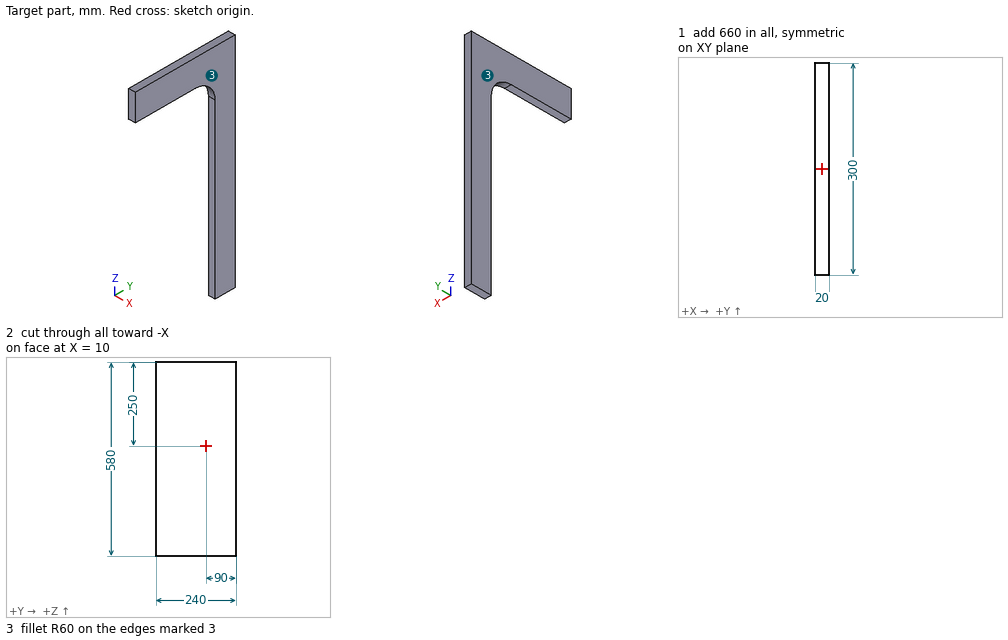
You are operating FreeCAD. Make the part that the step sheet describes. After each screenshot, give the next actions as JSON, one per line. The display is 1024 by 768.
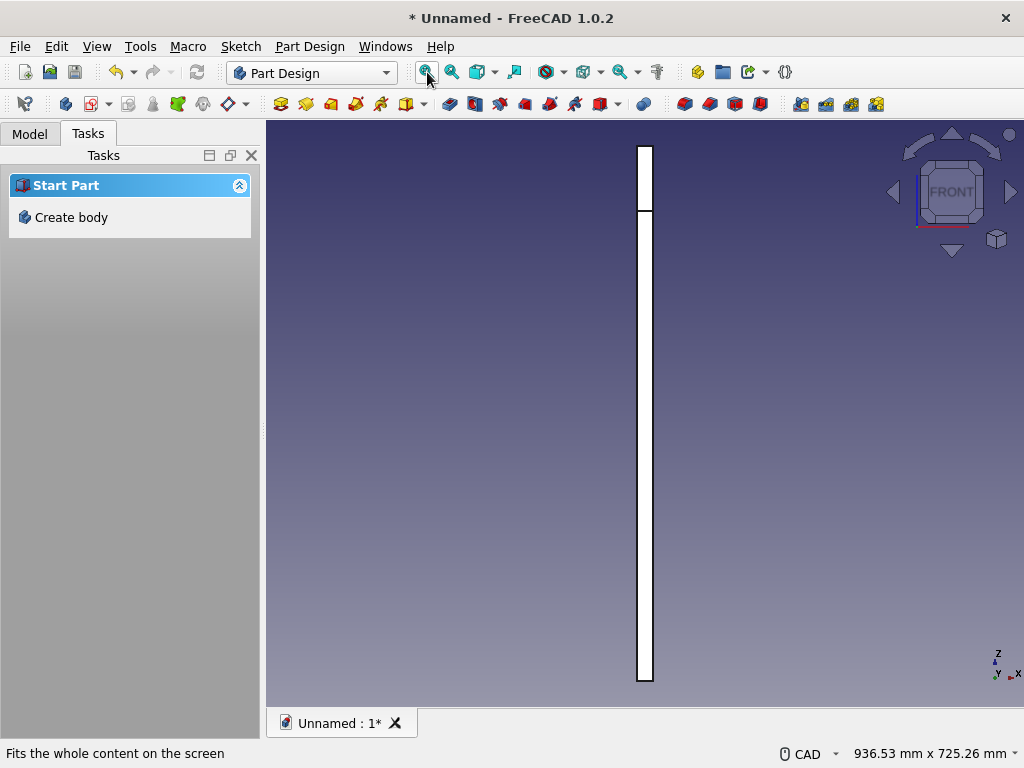
{"action": "key", "text": "3"}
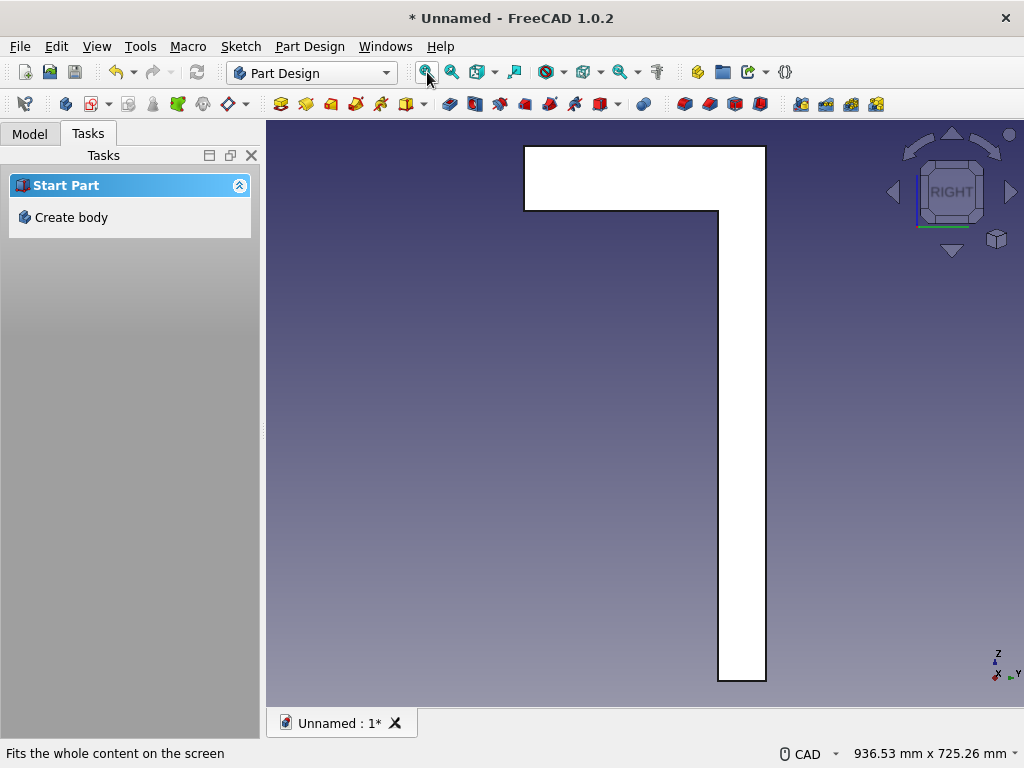
{"action": "scroll", "coordinate": [718, 210], "scroll_direction": "up", "scroll_amount": 5}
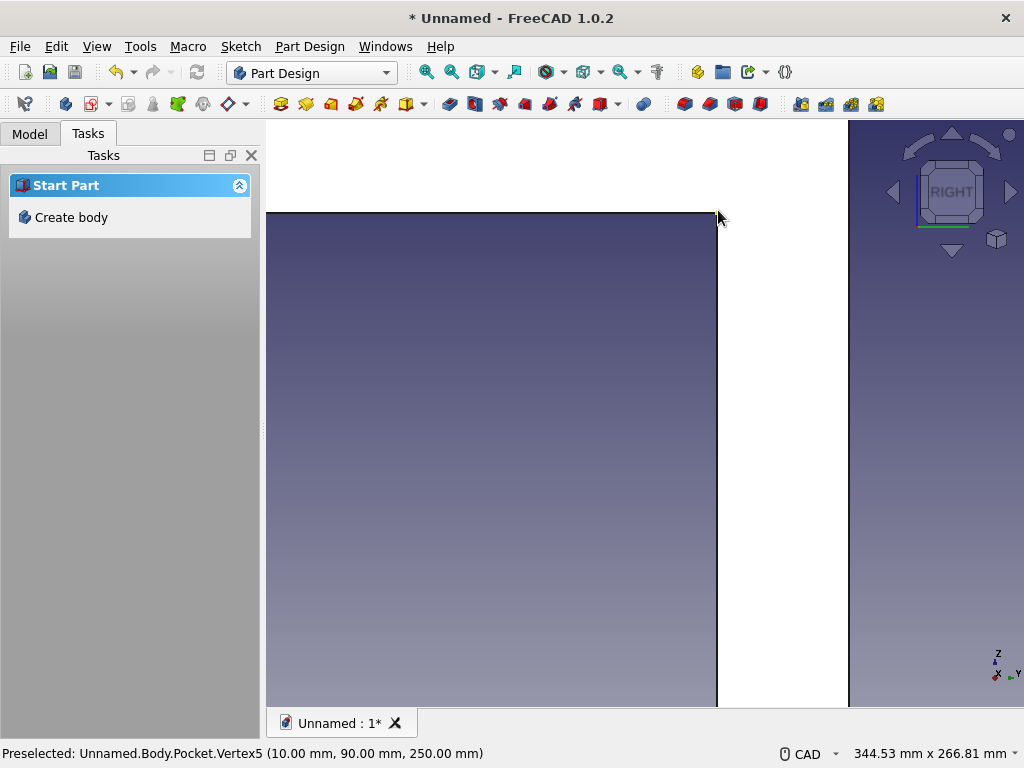
{"action": "left_click", "coordinate": [427, 72]}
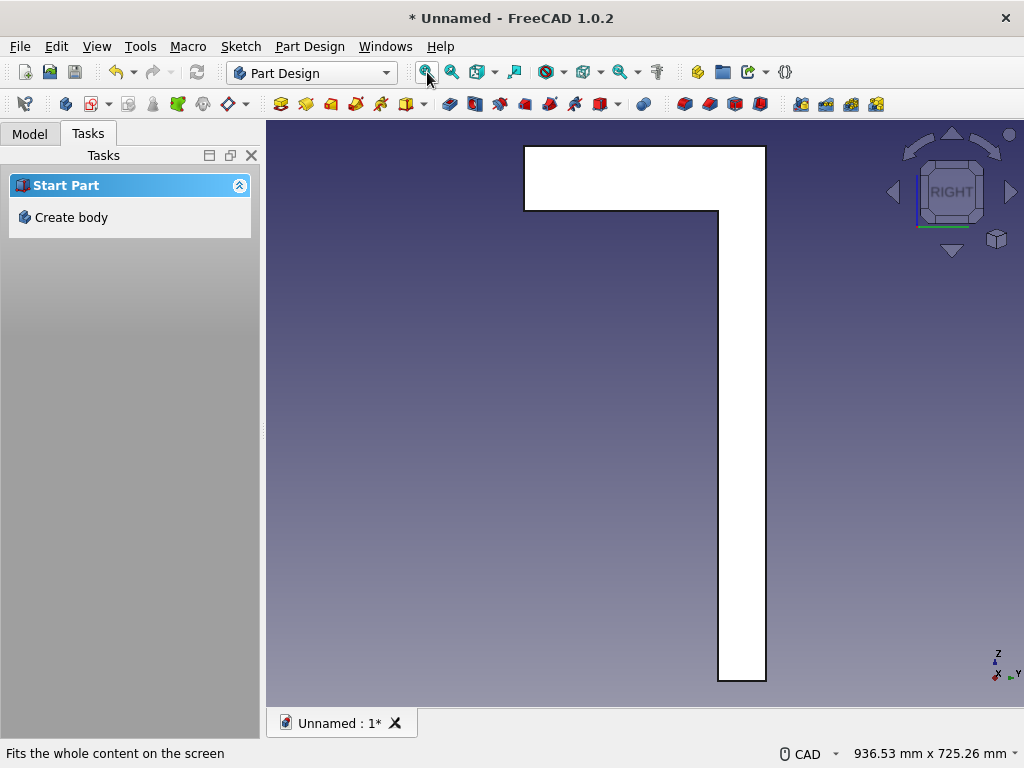
{"action": "key", "text": "5"}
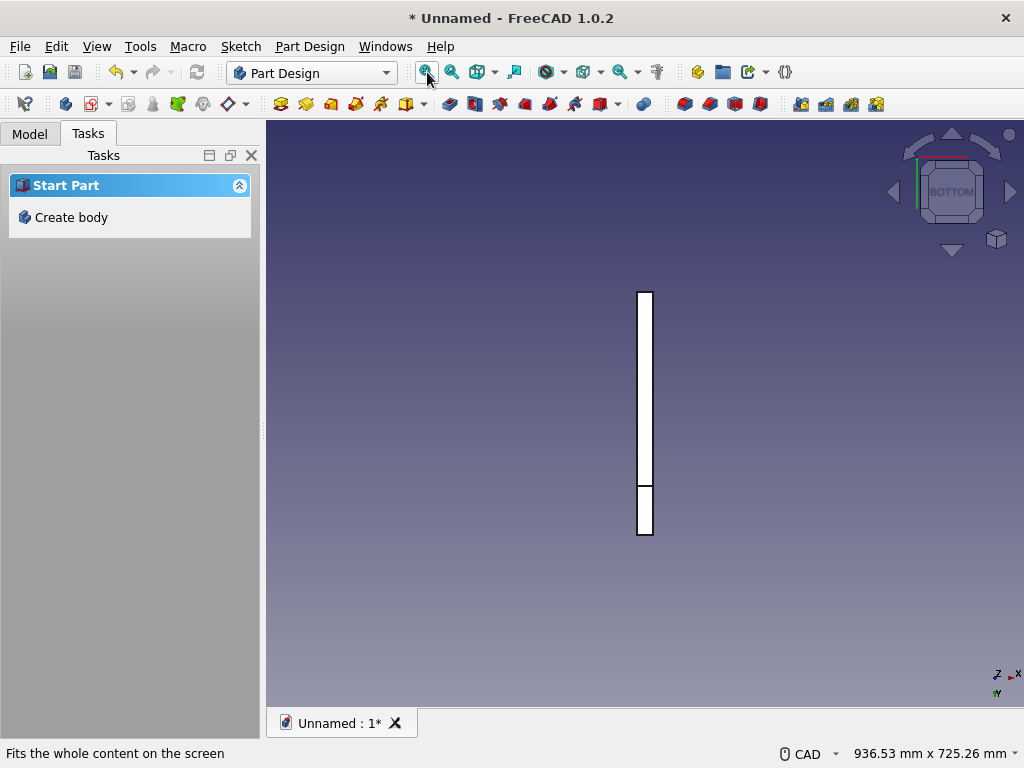
{"action": "left_click", "coordinate": [427, 72]}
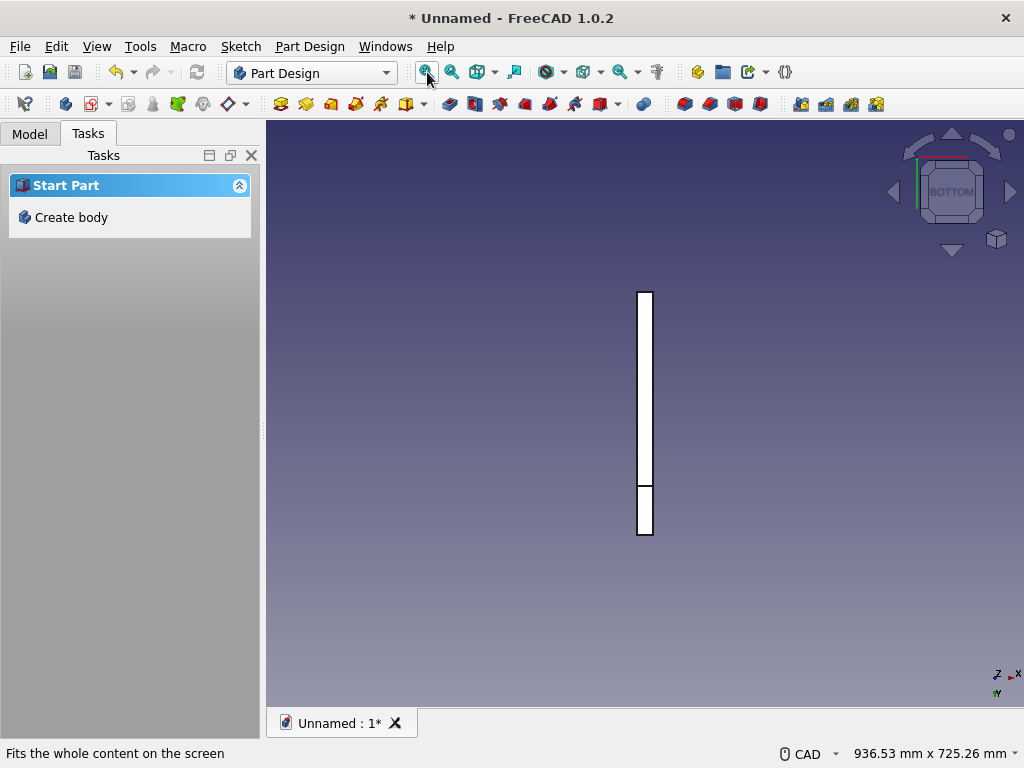
{"action": "scroll", "coordinate": [645, 485], "scroll_direction": "up", "scroll_amount": 5}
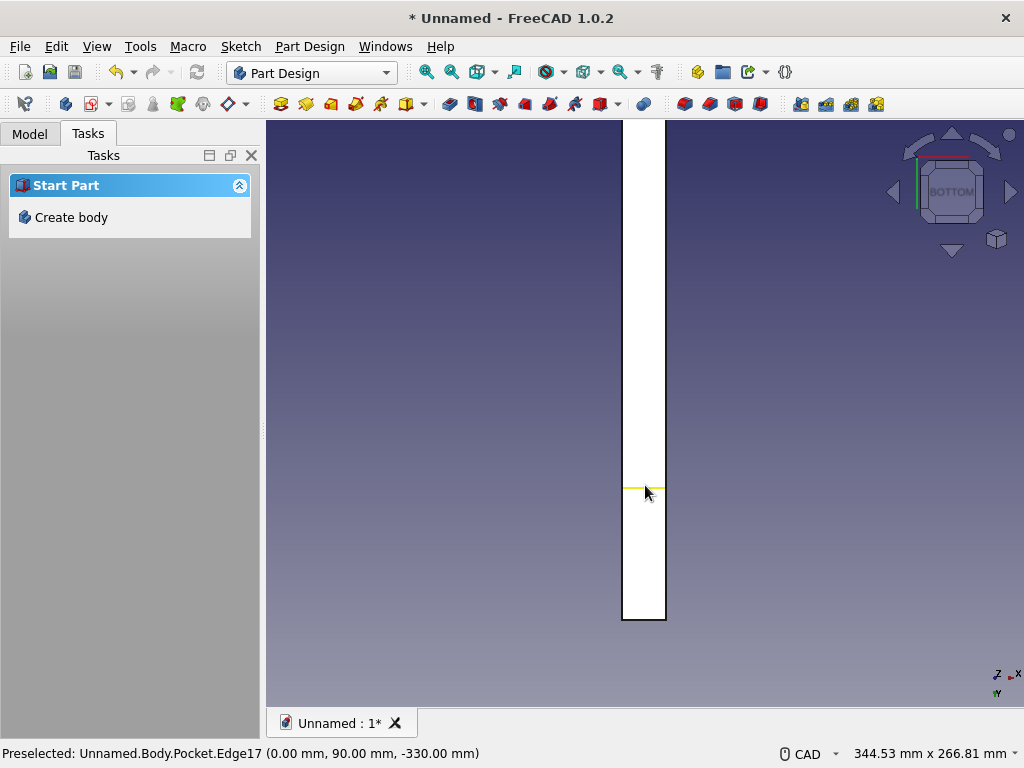
{"action": "left_click", "coordinate": [427, 72]}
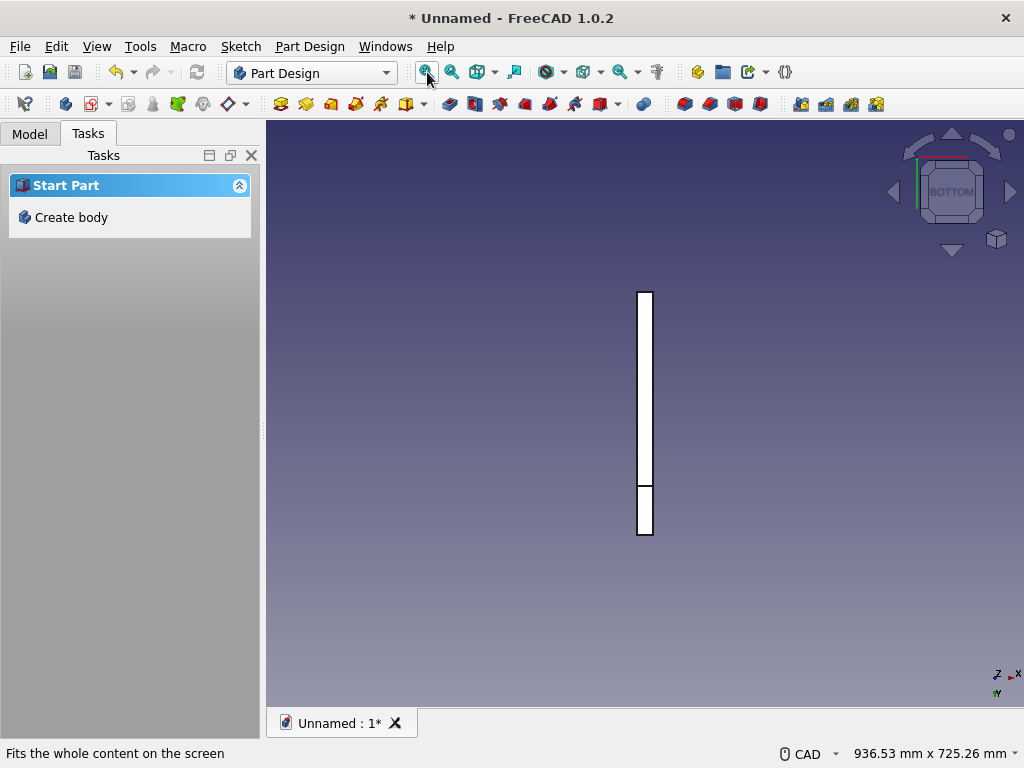
{"action": "key", "text": "4"}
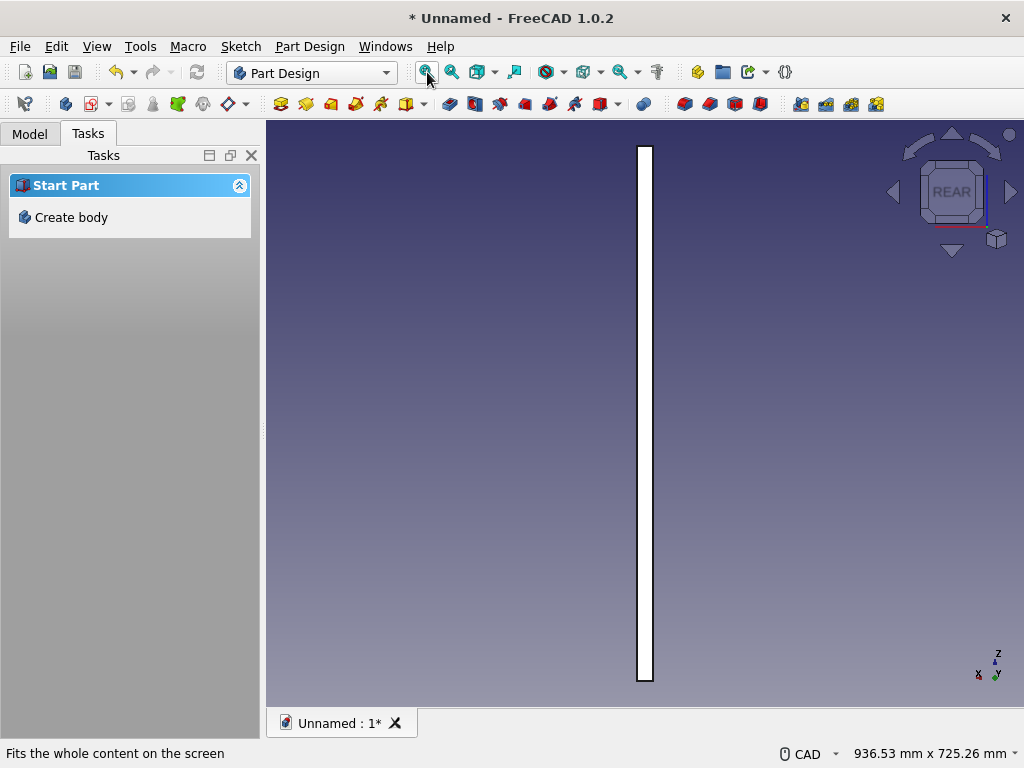
{"action": "scroll", "coordinate": [645, 210], "scroll_direction": "up", "scroll_amount": 5}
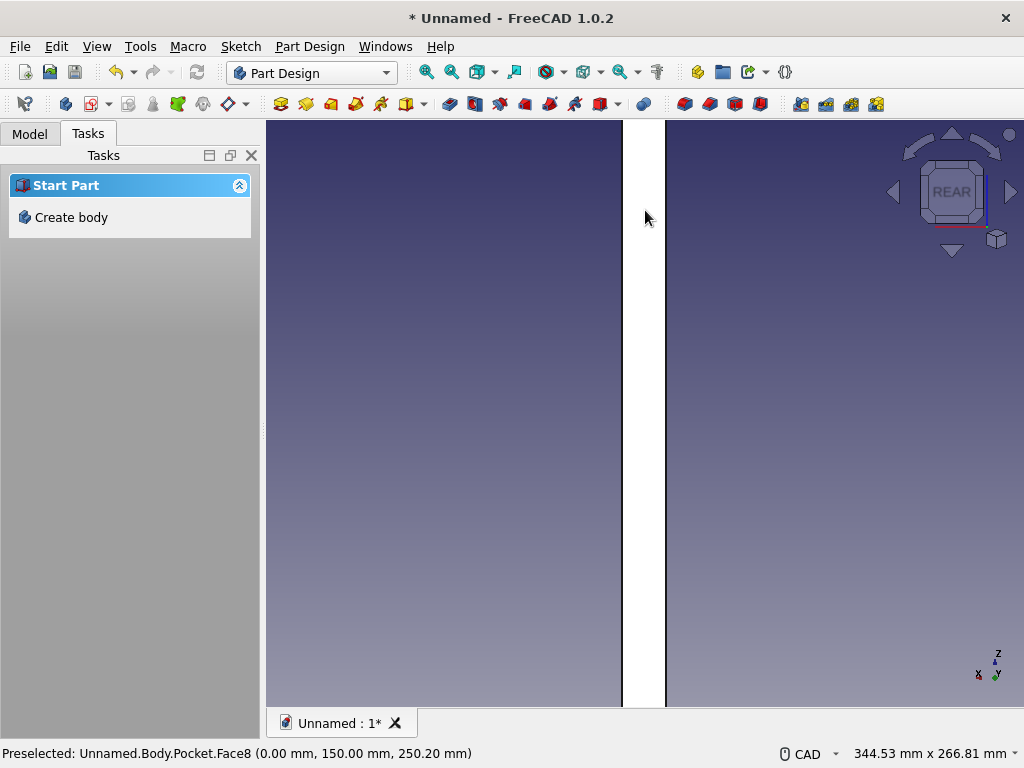
{"action": "left_click", "coordinate": [427, 72]}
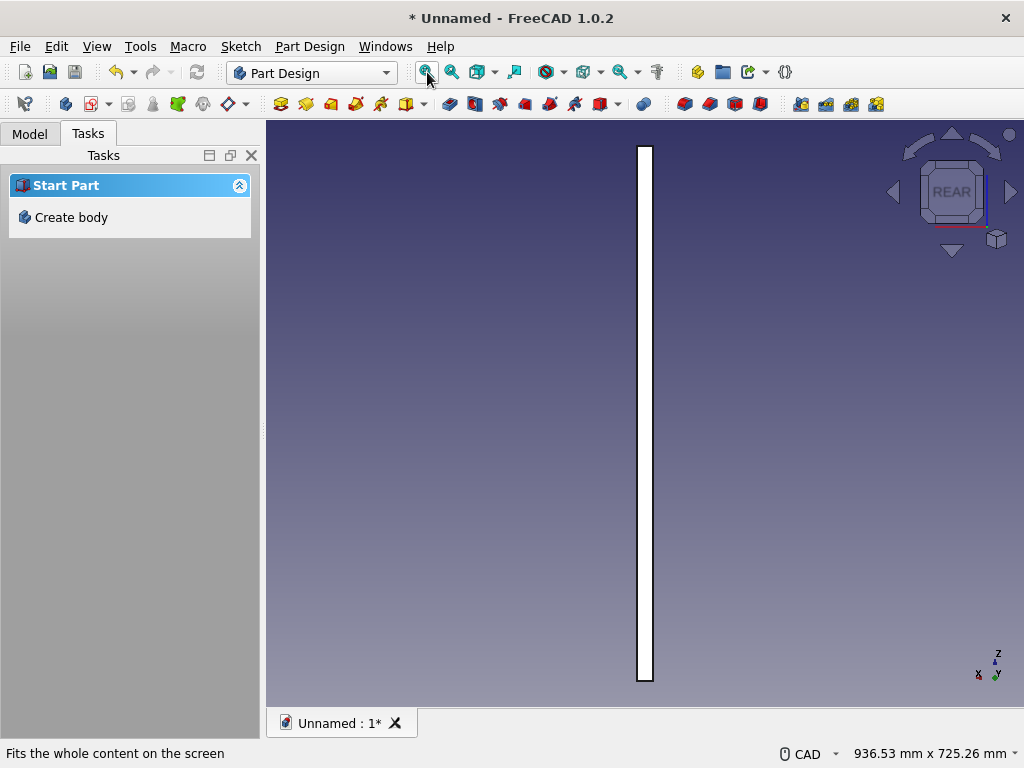
{"action": "key", "text": "6"}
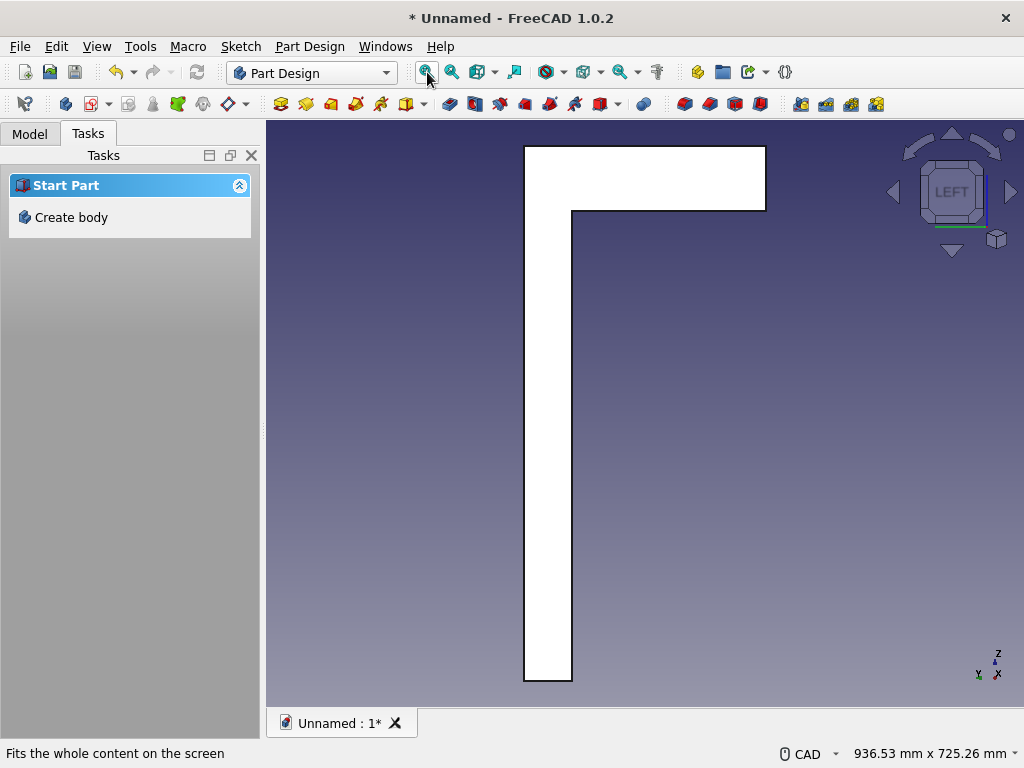
{"action": "scroll", "coordinate": [572, 210], "scroll_direction": "up", "scroll_amount": 5}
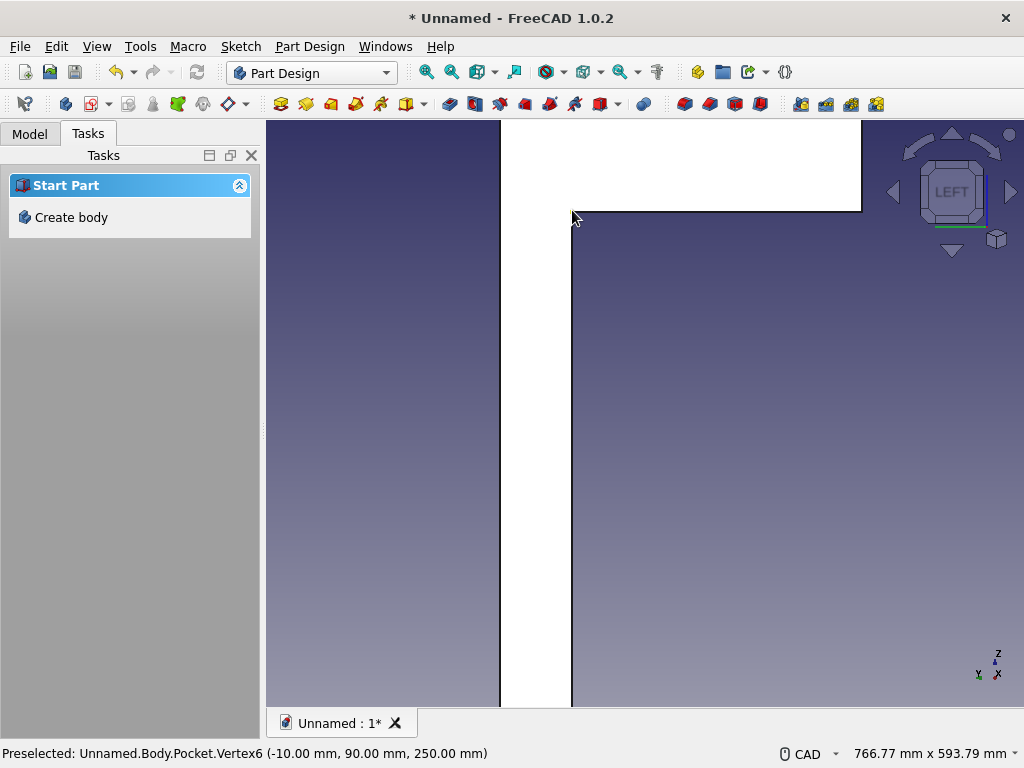
{"action": "left_click", "coordinate": [427, 72]}